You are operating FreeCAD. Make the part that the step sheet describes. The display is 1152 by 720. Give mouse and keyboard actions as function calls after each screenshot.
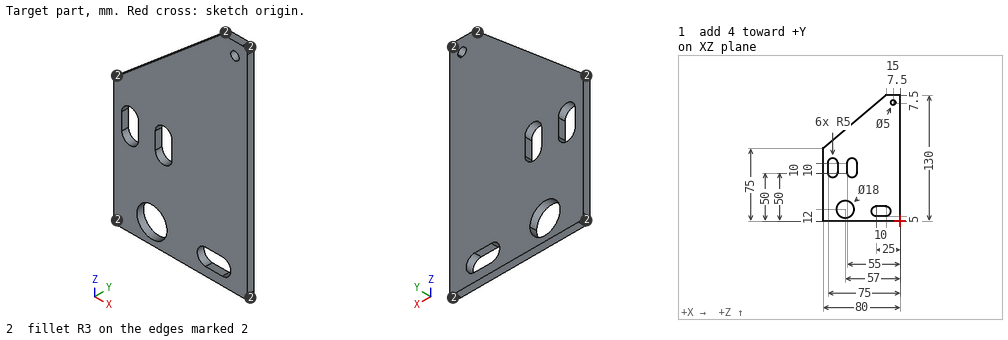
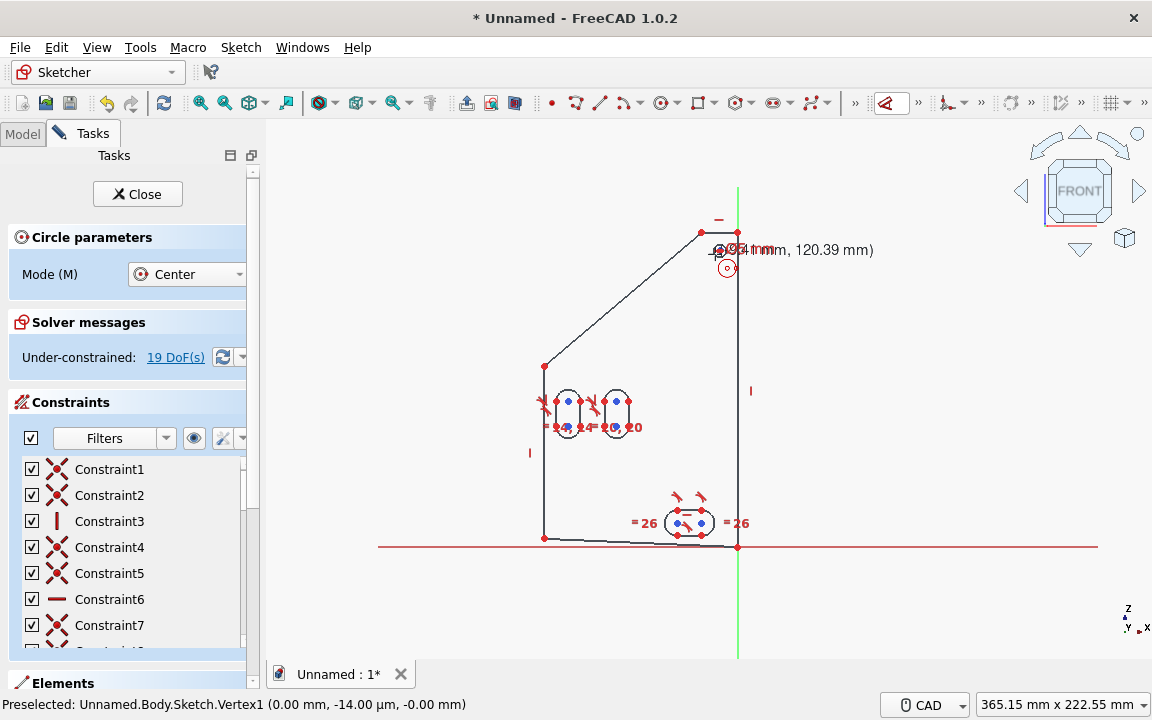
click(600, 518)
move(615, 503)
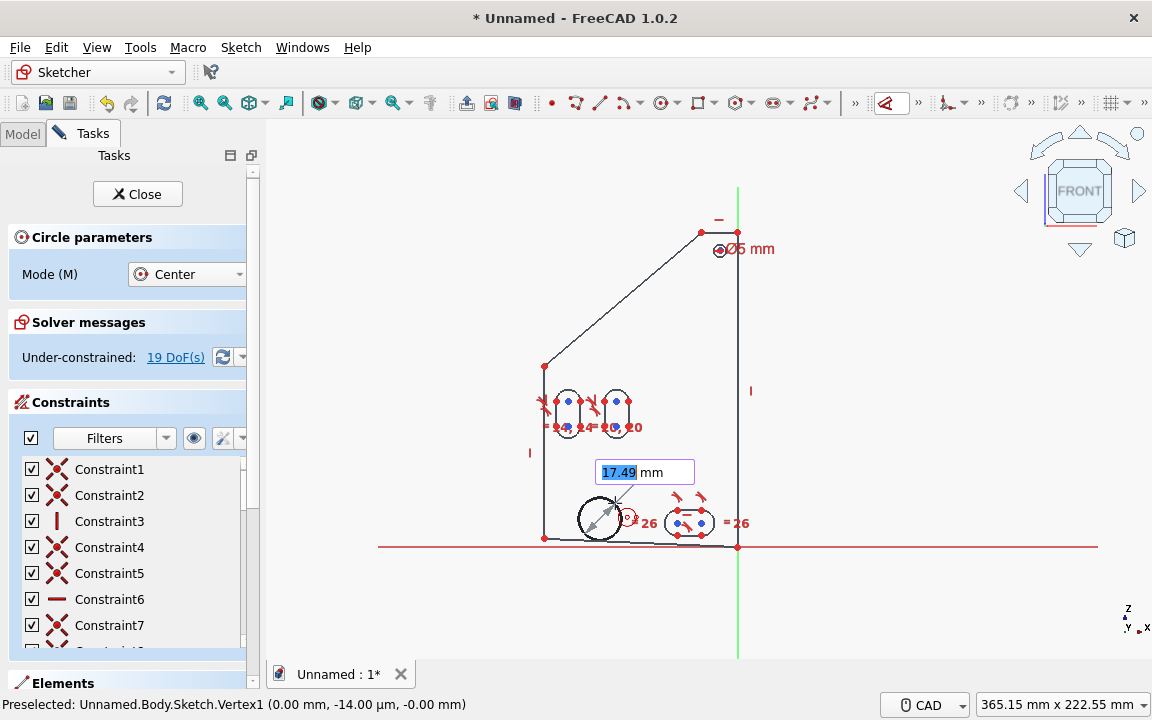
text(18)
key(Return)
key(Escape)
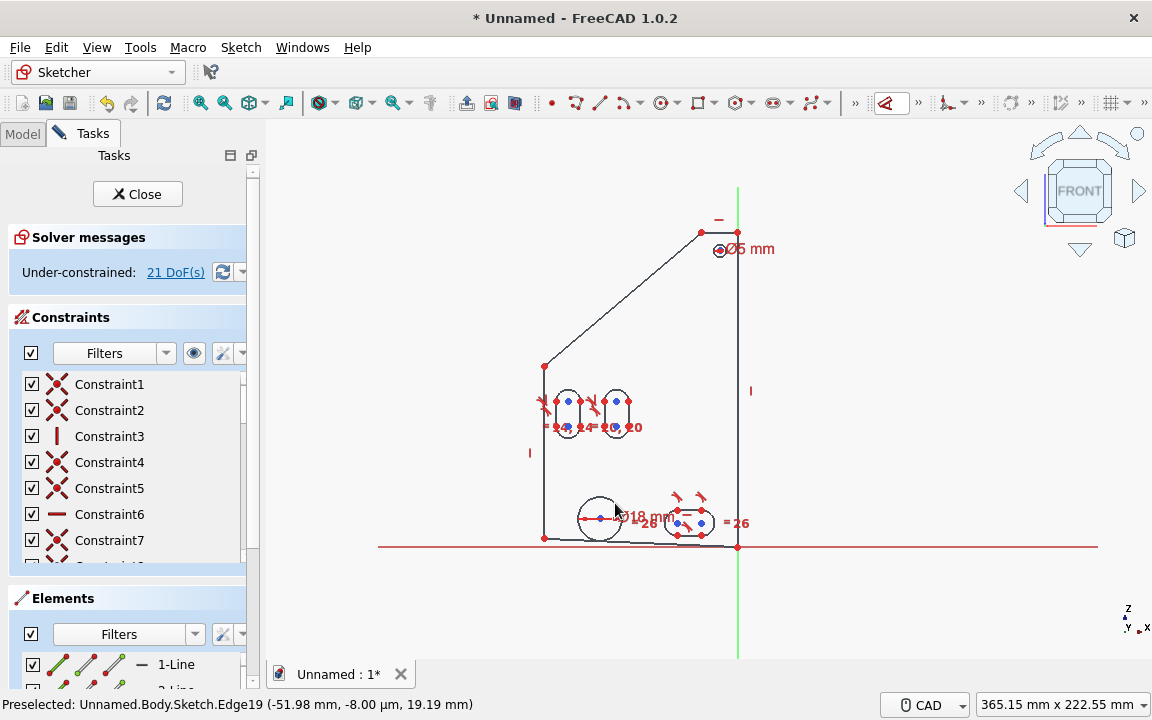
click(660, 544)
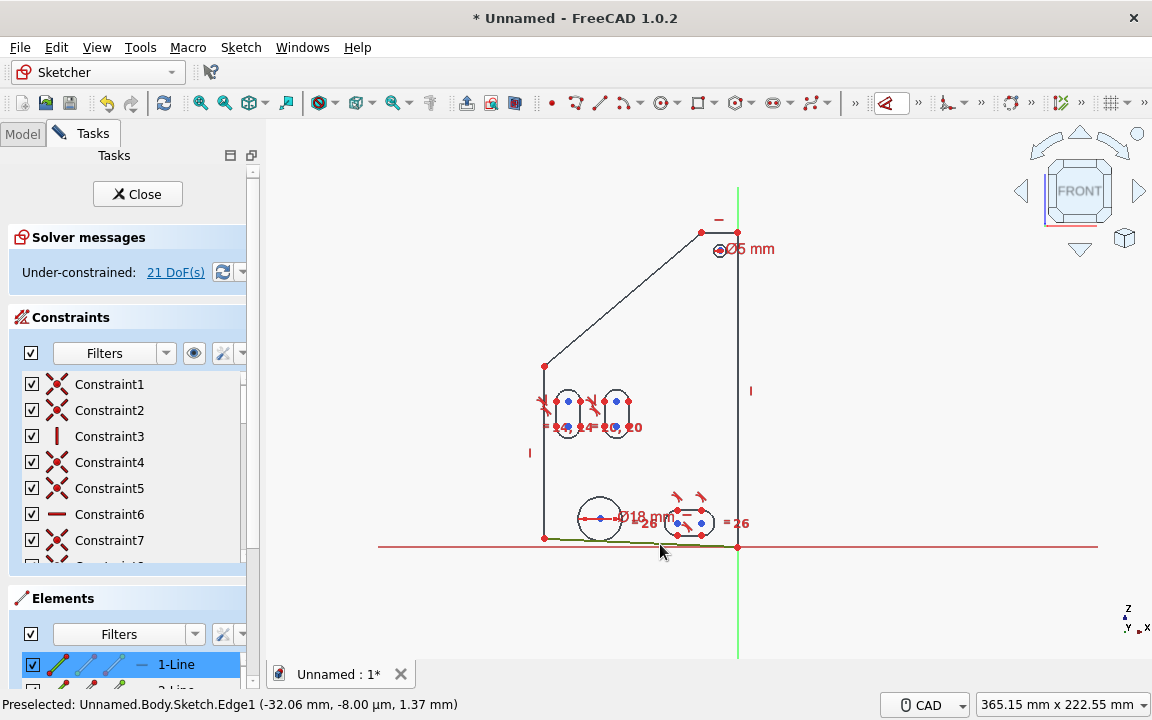
key(h)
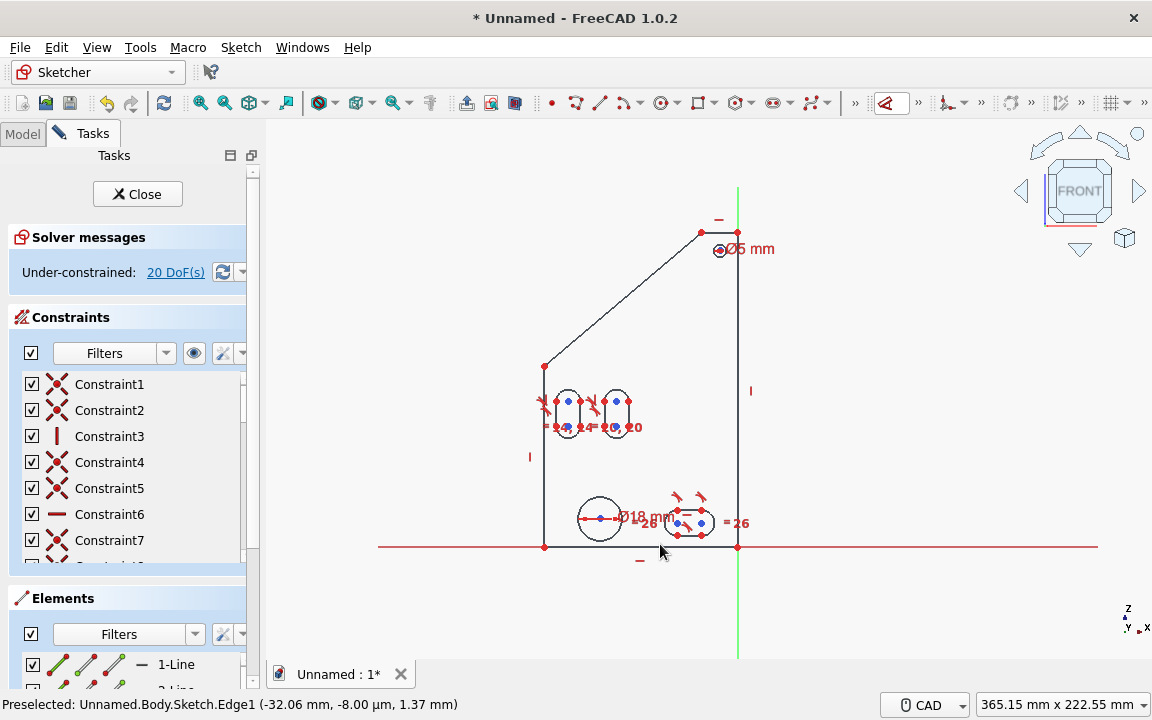
scroll(561, 436, up, 2)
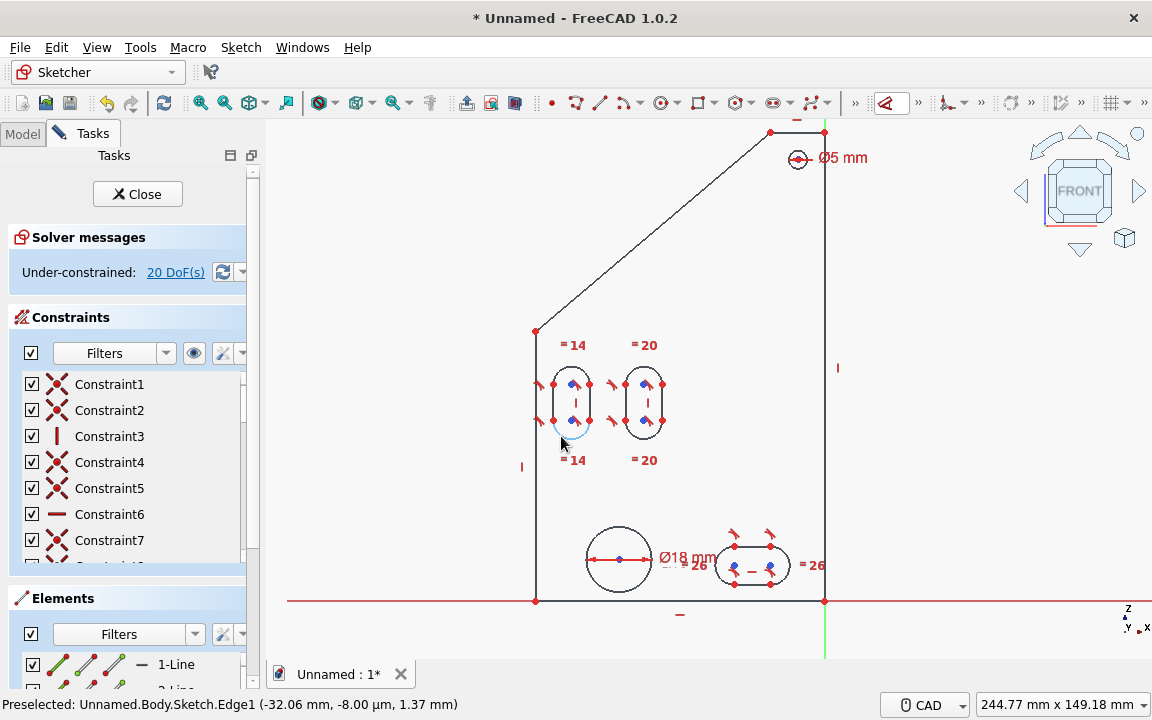
click(561, 436)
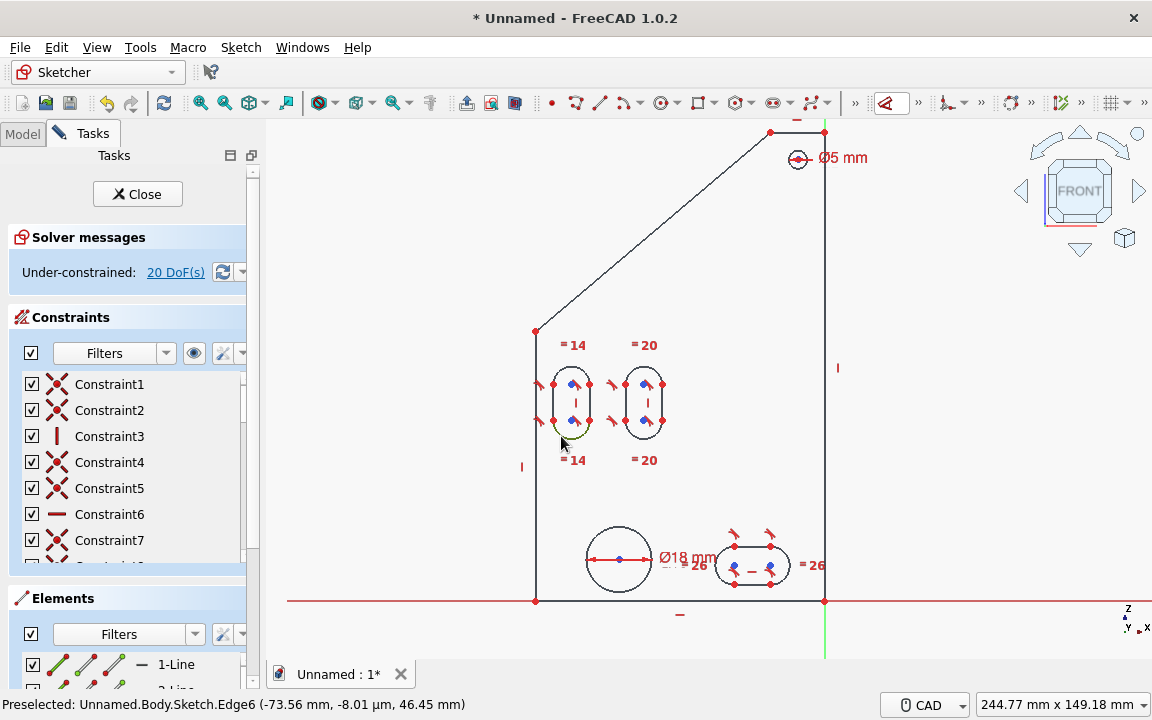
click(633, 436)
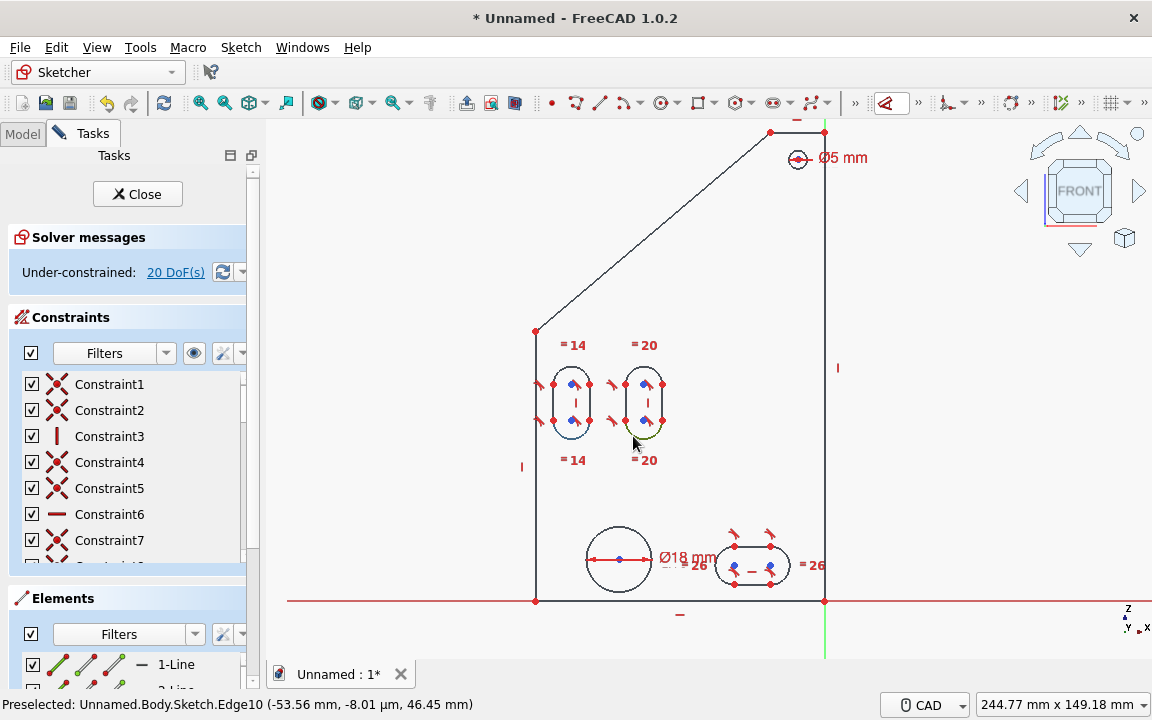
click(719, 555)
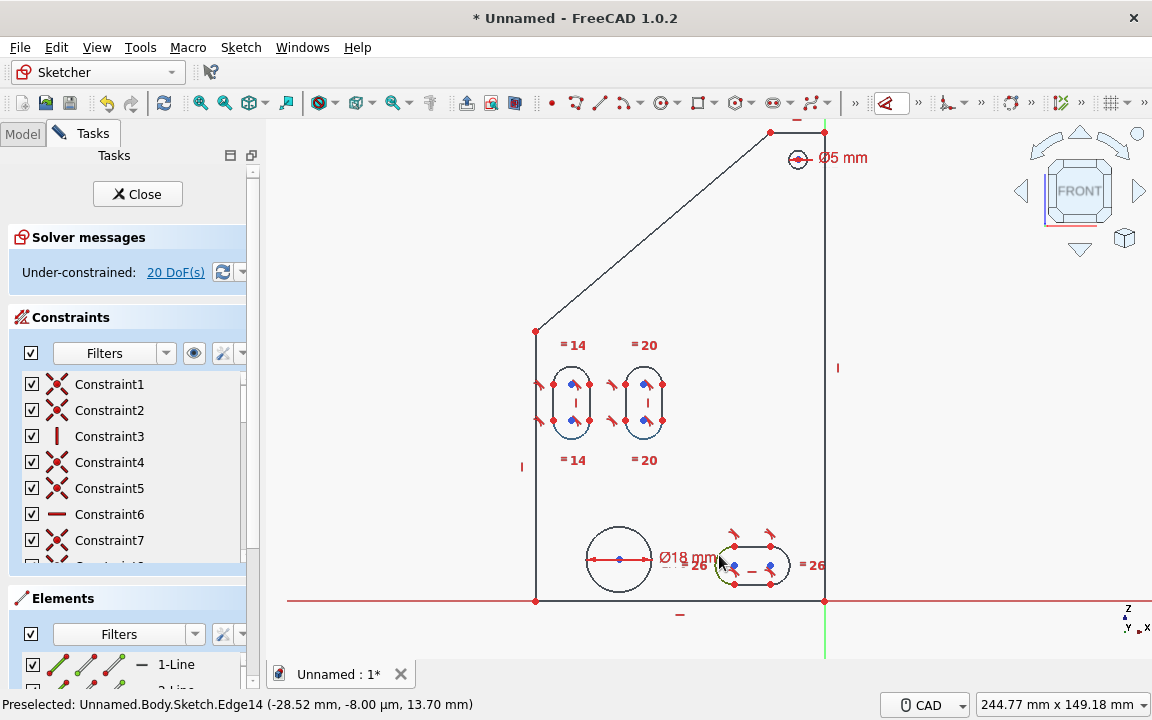
key(e)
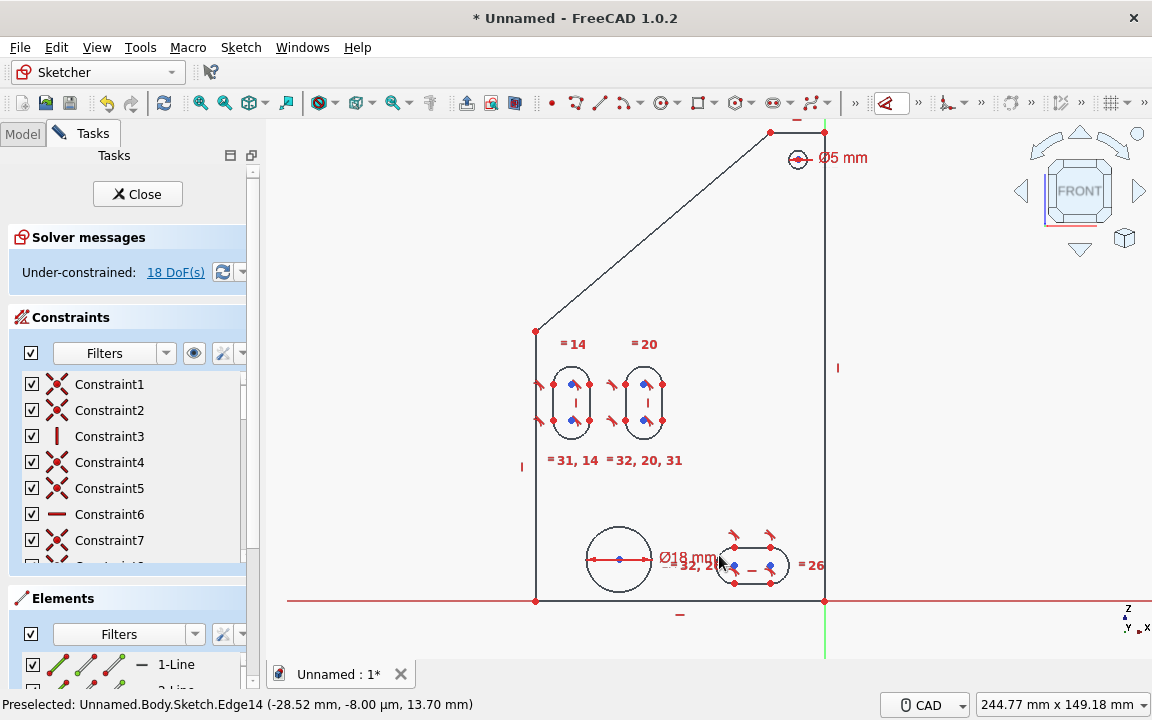
click(886, 104)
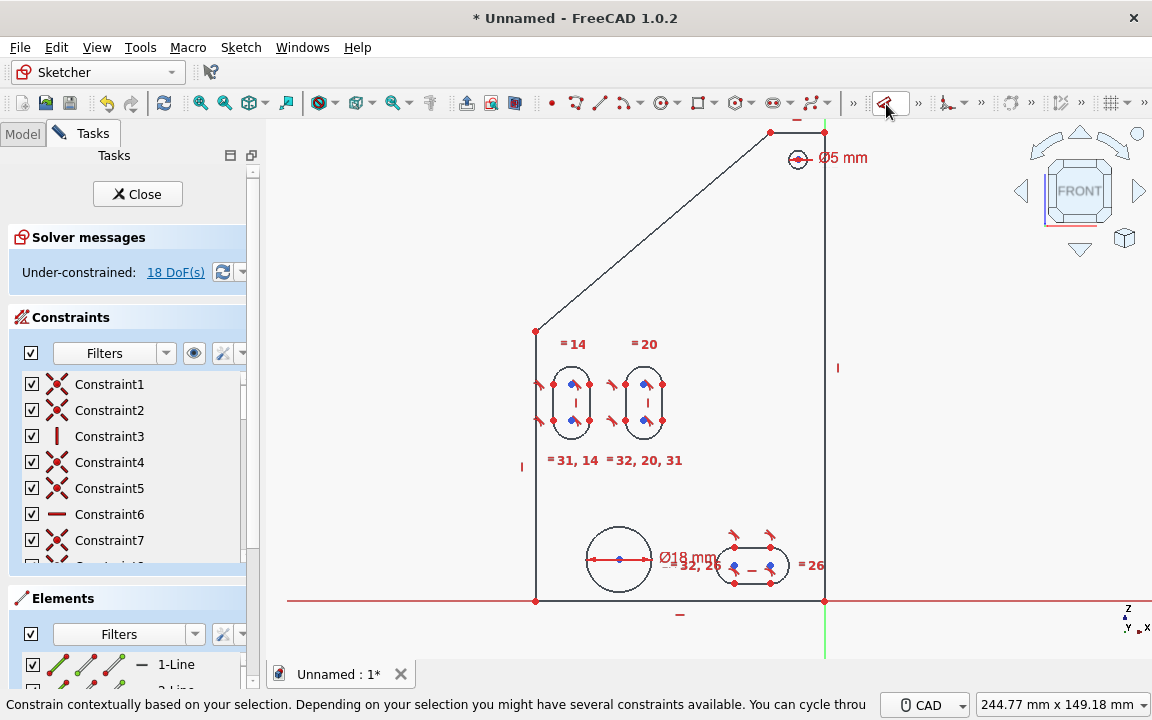
scroll(561, 436, up, 4)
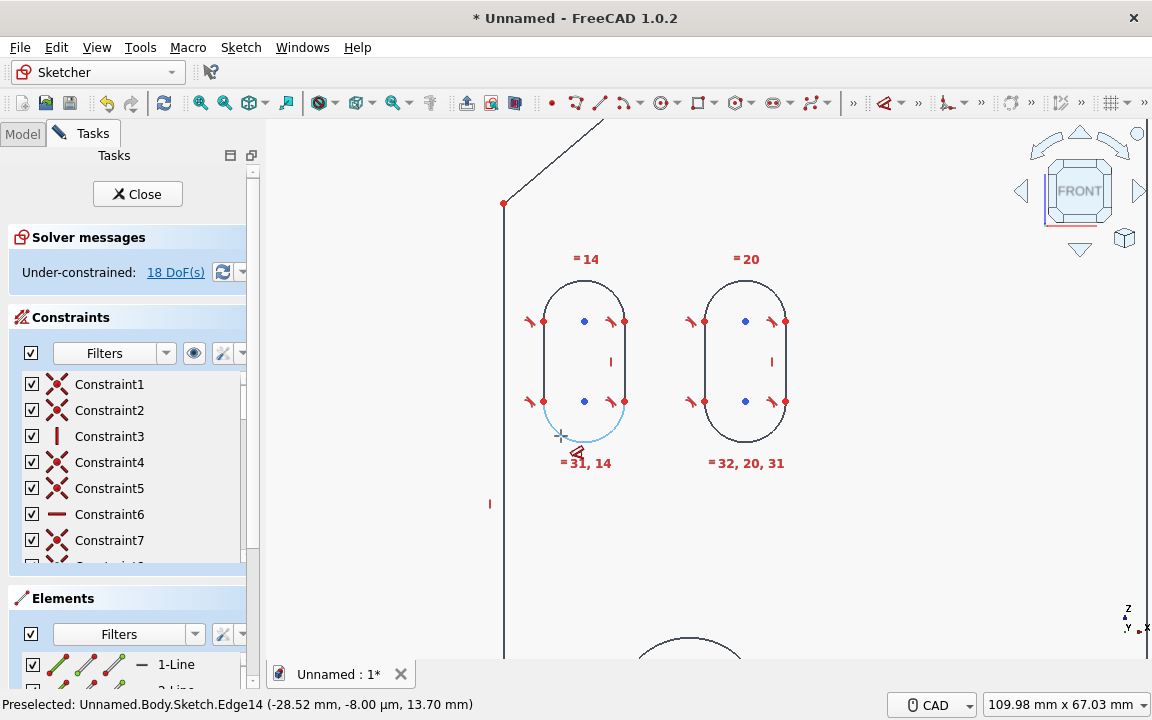
click(560, 435)
click(541, 461)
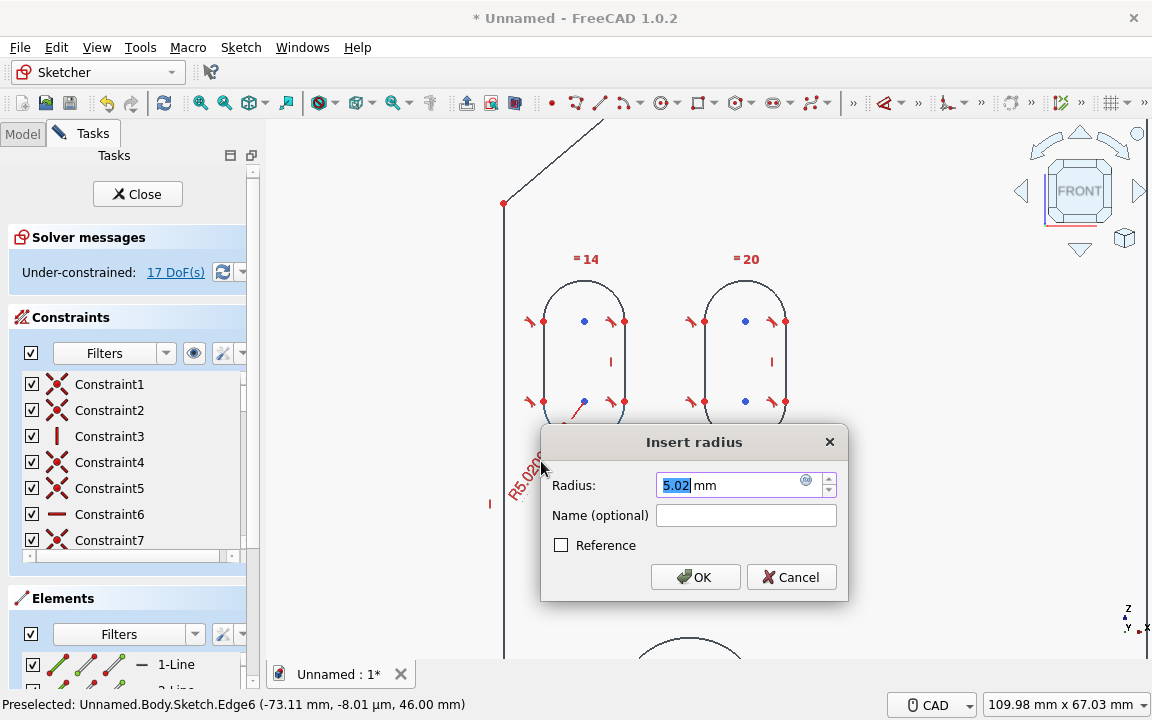
text(5)
key(Return)